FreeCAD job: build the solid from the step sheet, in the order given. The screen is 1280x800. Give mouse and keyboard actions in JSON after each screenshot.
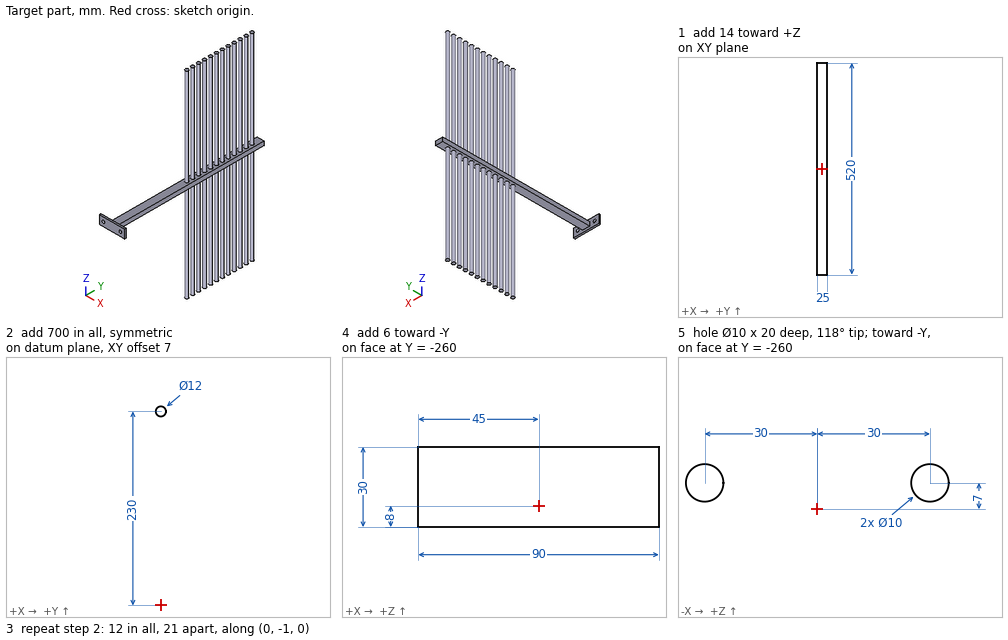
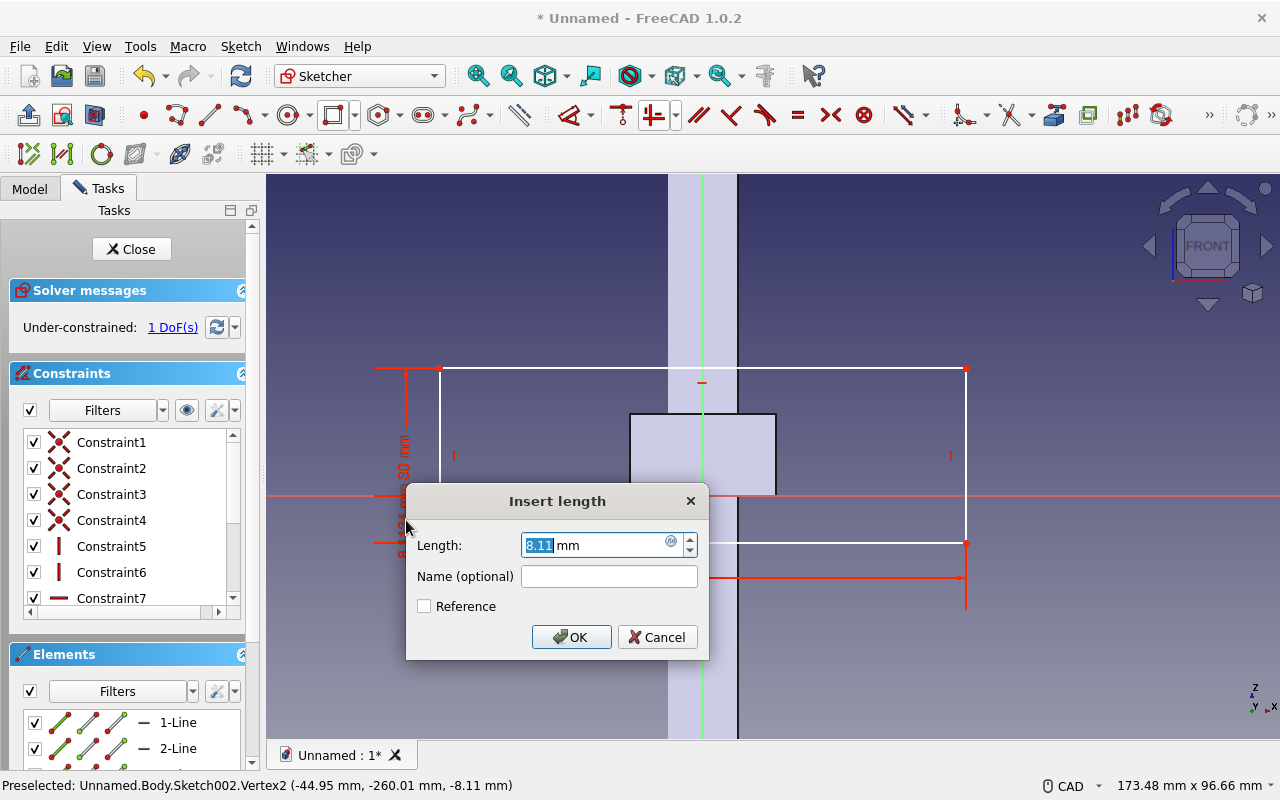
{"action": "type", "text": "8"}
{"action": "key", "text": "Return"}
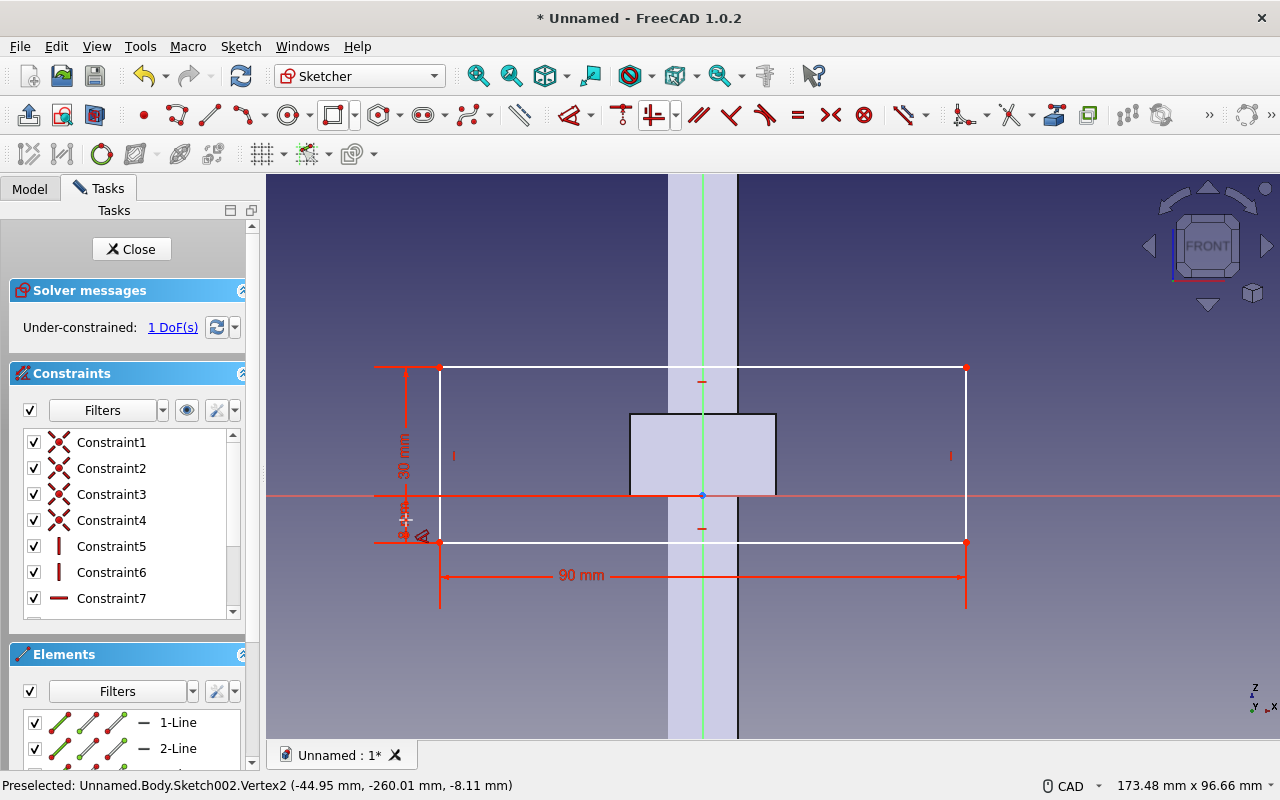
{"action": "left_click", "coordinate": [440, 367]}
{"action": "left_click", "coordinate": [571, 333]}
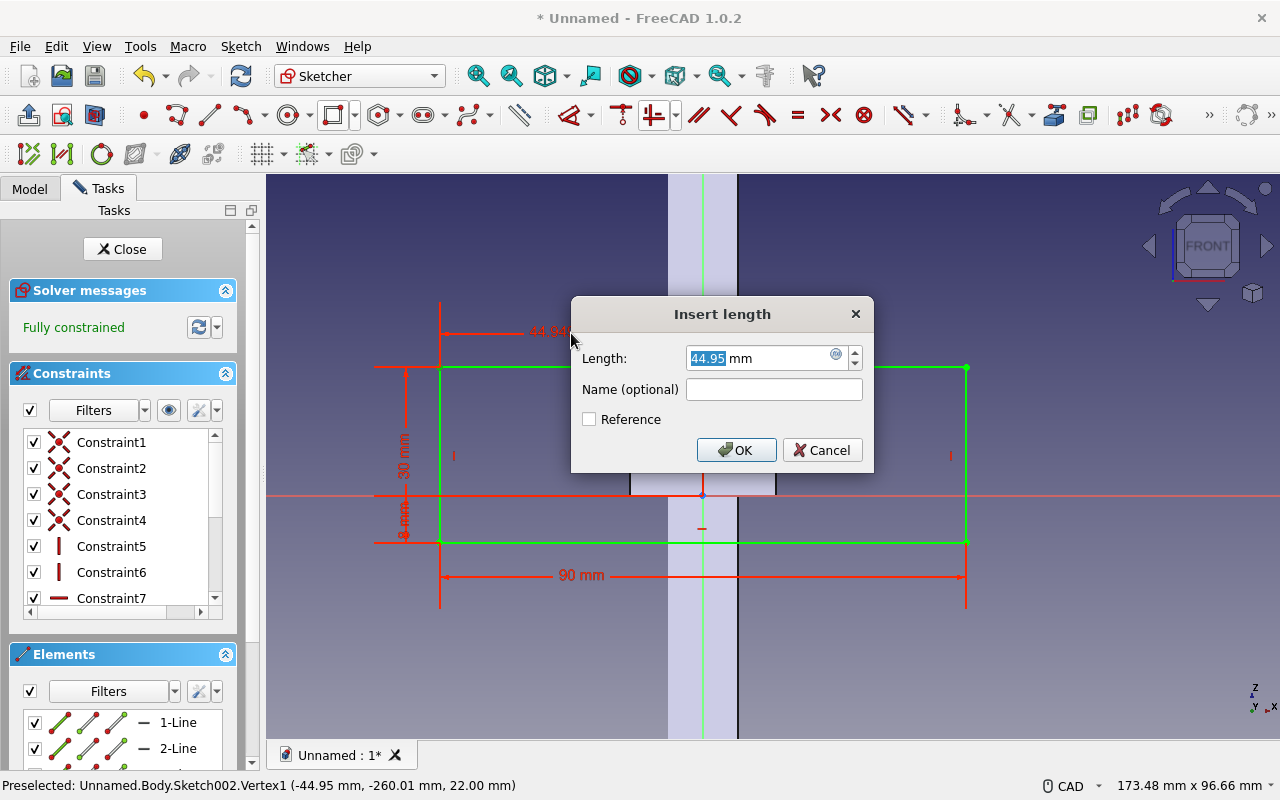
{"action": "type", "text": "45"}
{"action": "key", "text": "Return"}
{"action": "key", "text": "Escape"}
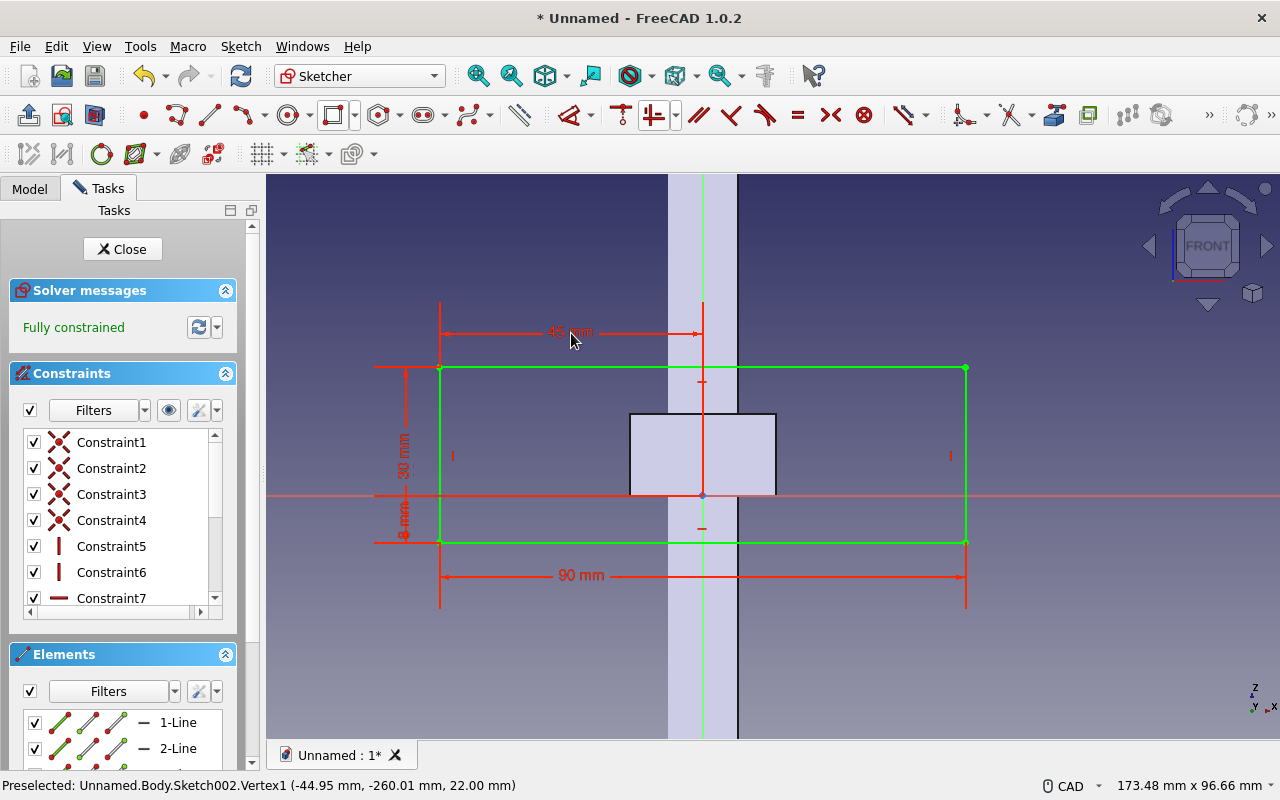
{"action": "left_click", "coordinate": [123, 249]}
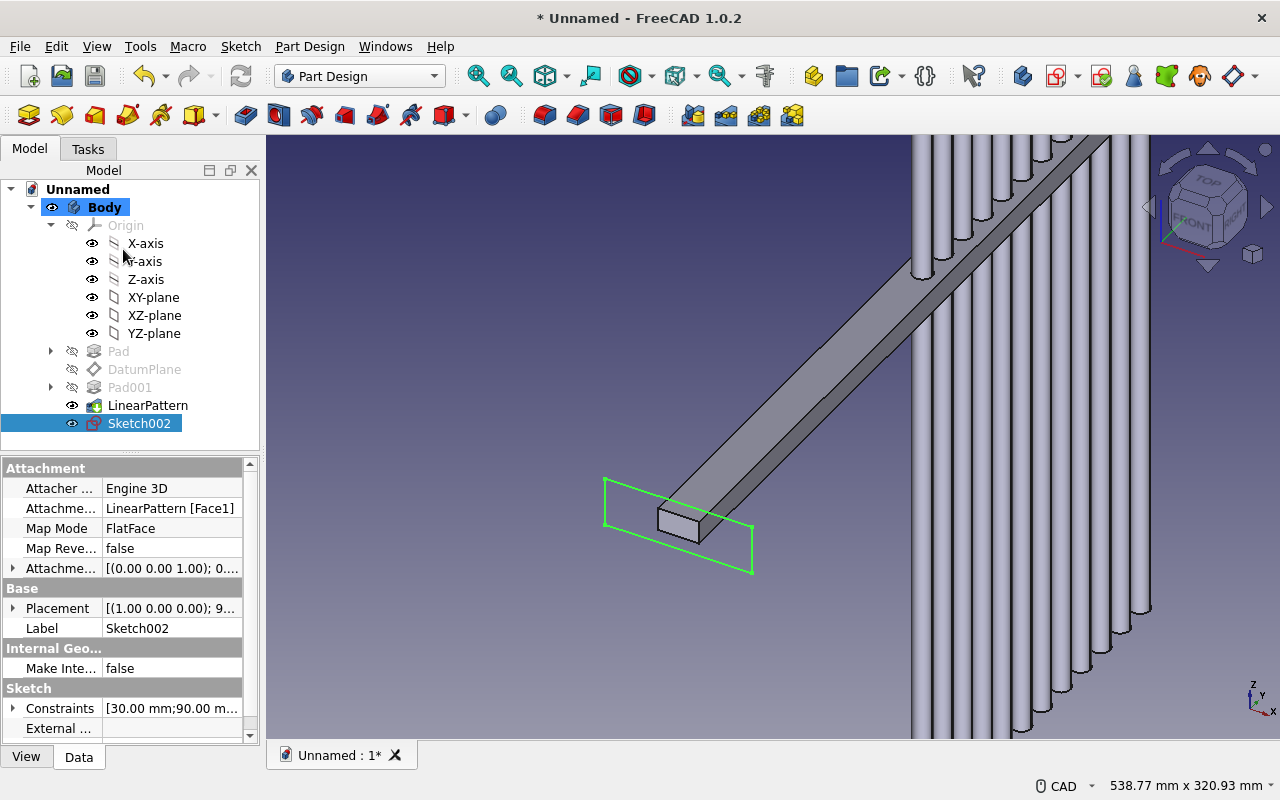
{"action": "left_click", "coordinate": [29, 116]}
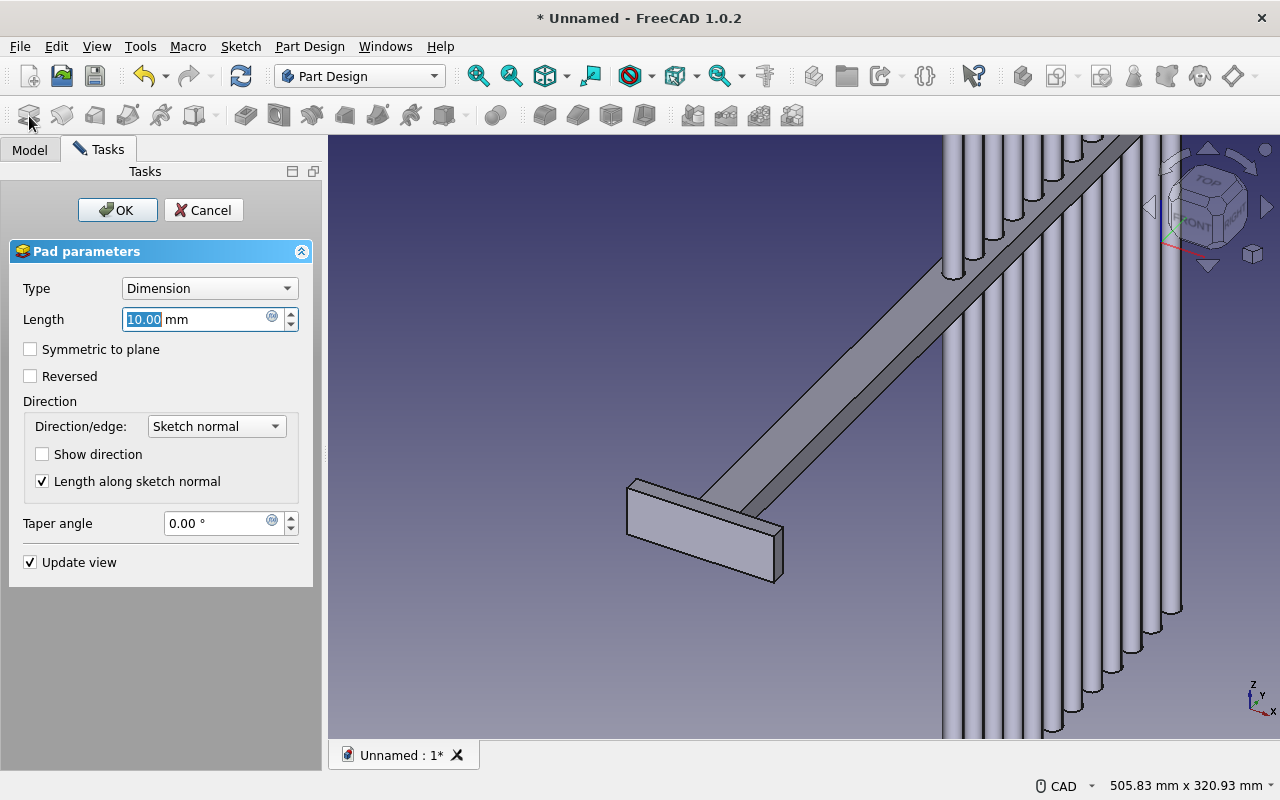
{"action": "type", "text": "6"}
{"action": "key", "text": "Tab"}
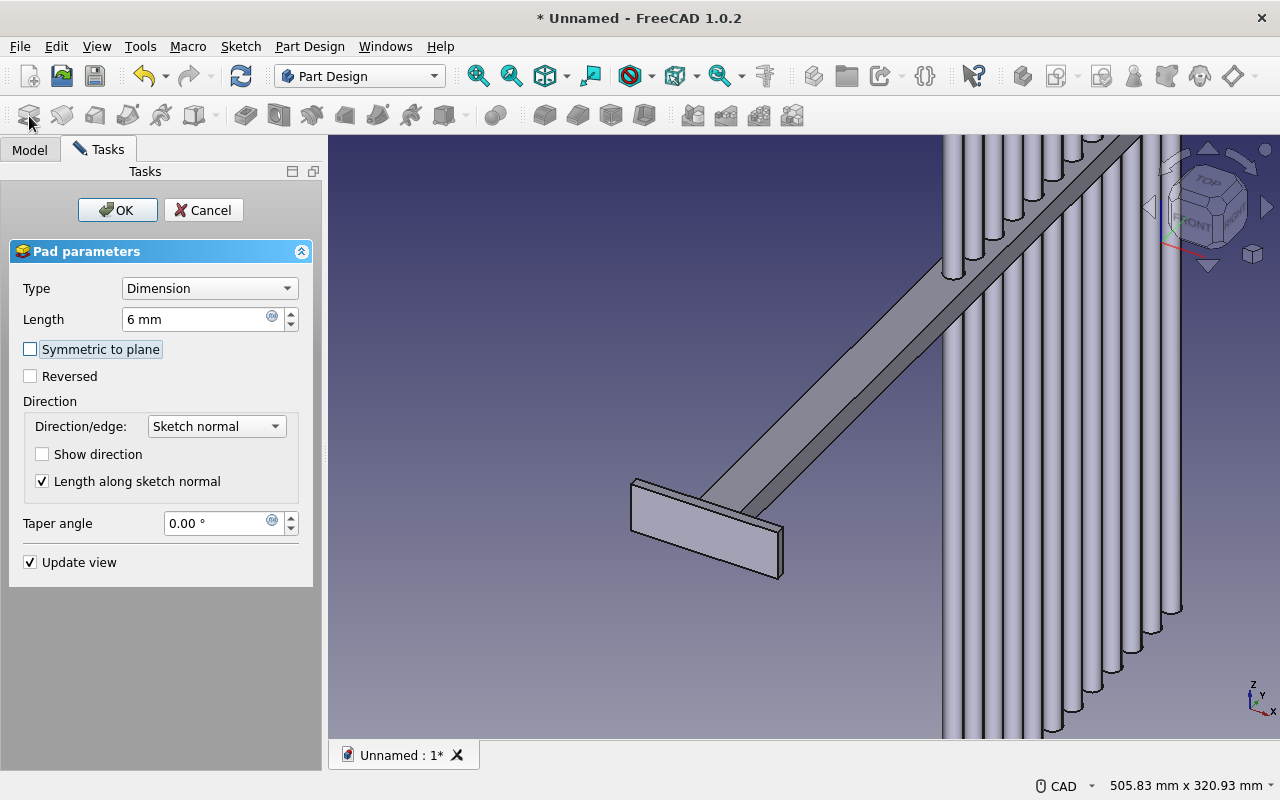
{"action": "left_click", "coordinate": [118, 210]}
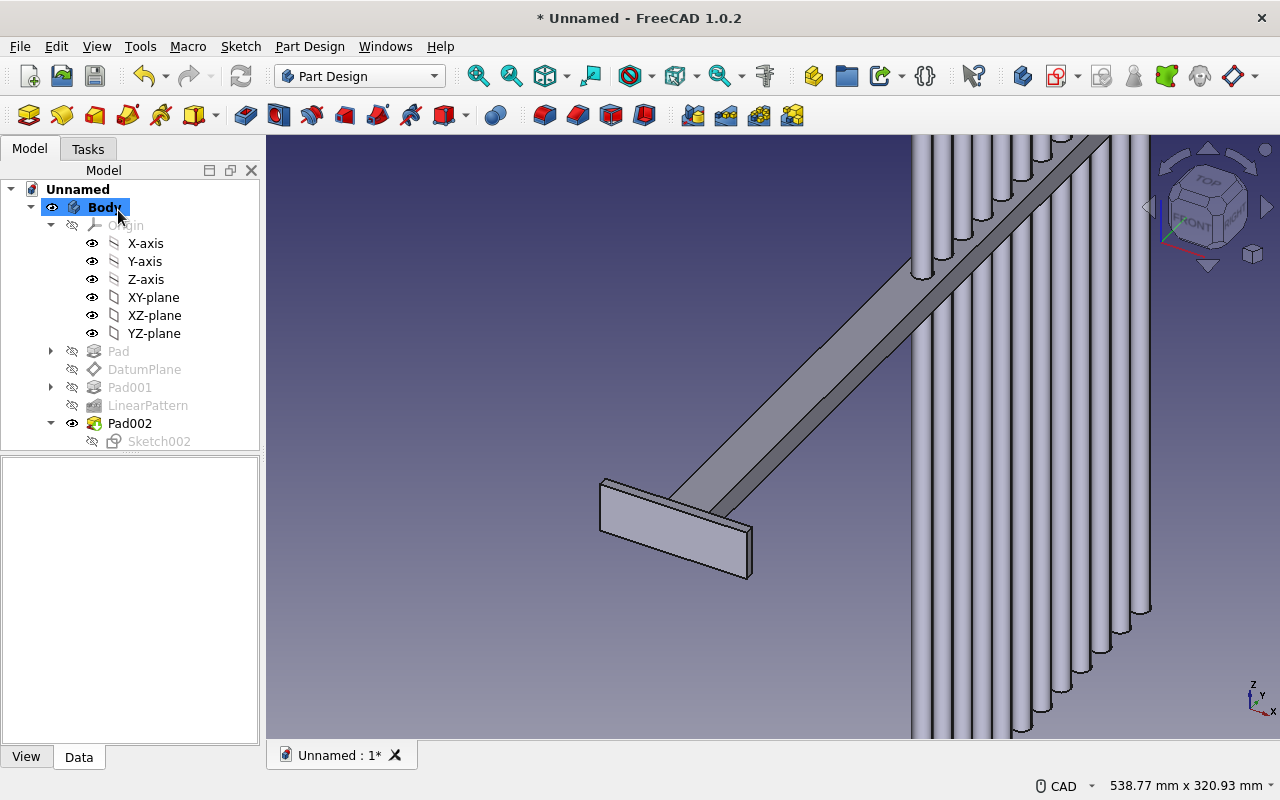
{"action": "left_click", "coordinate": [479, 76]}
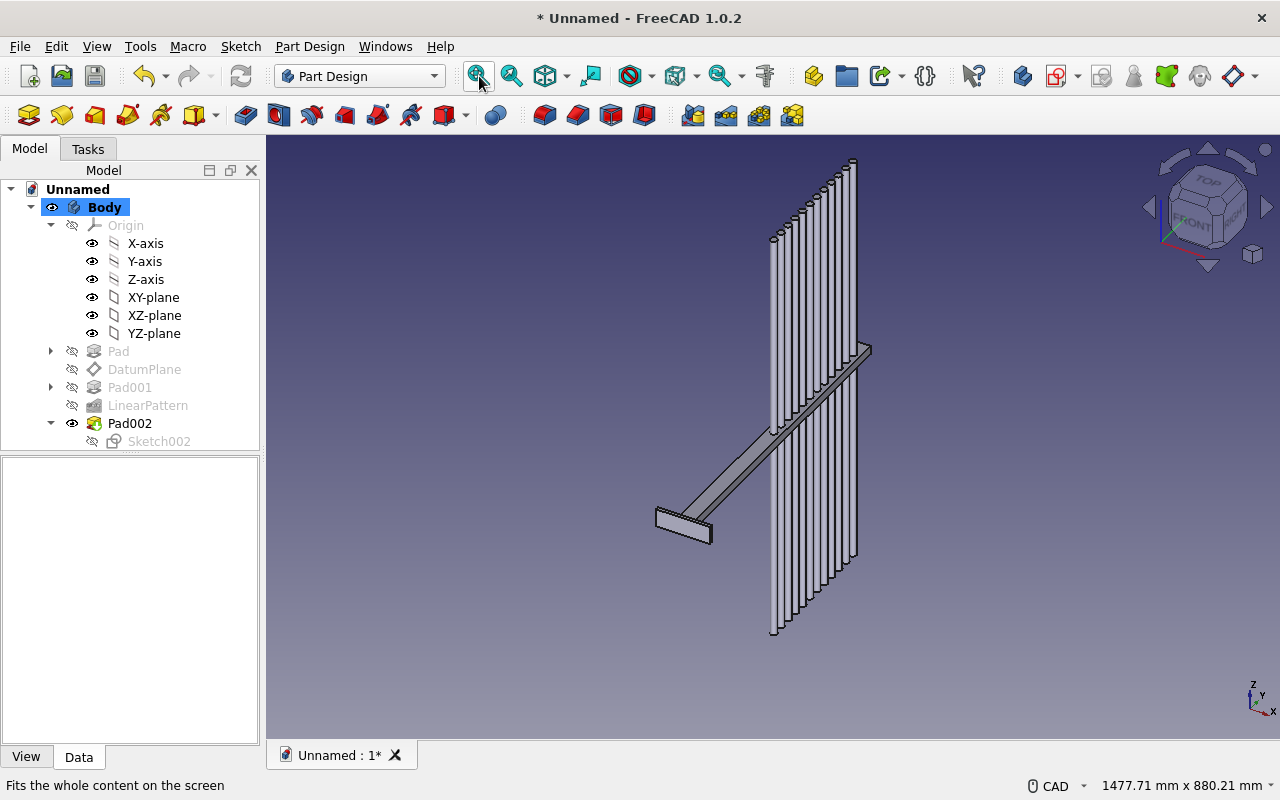
{"action": "key", "text": "4"}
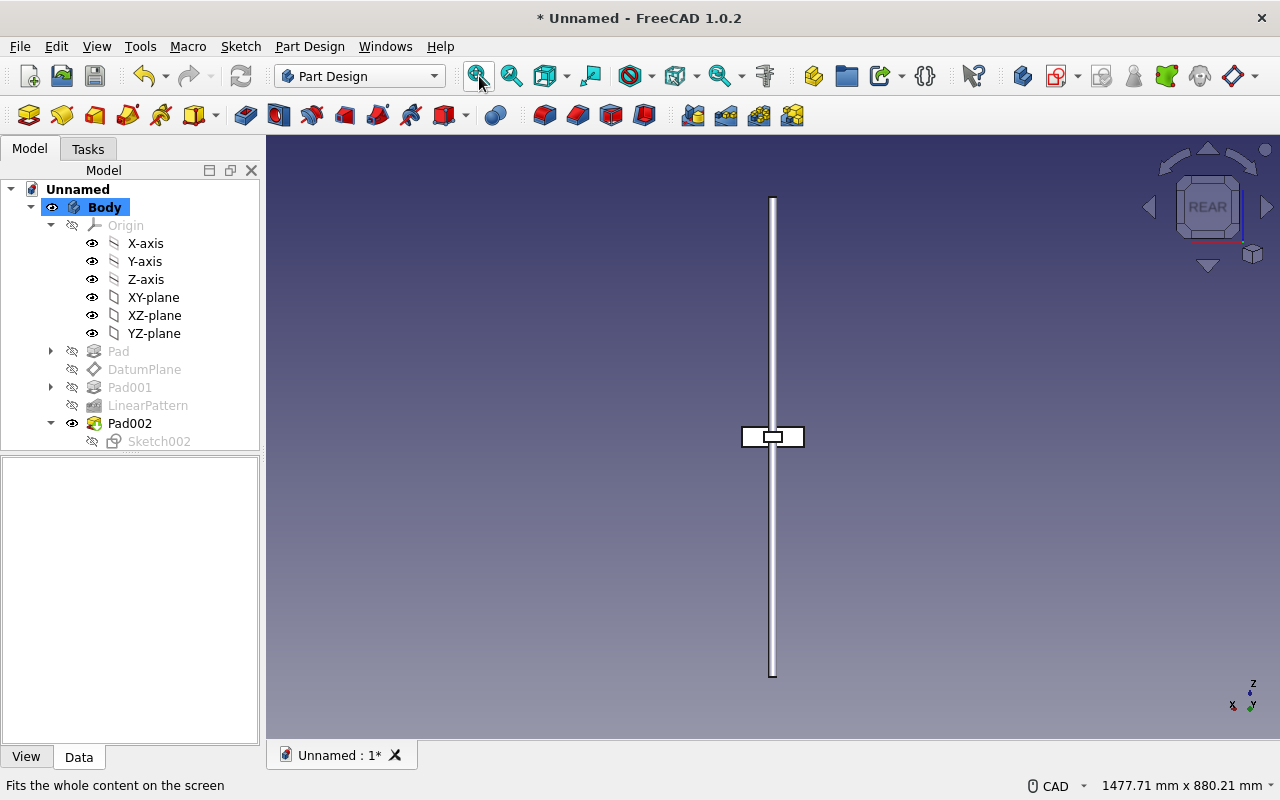
{"action": "left_click", "coordinate": [791, 436]}